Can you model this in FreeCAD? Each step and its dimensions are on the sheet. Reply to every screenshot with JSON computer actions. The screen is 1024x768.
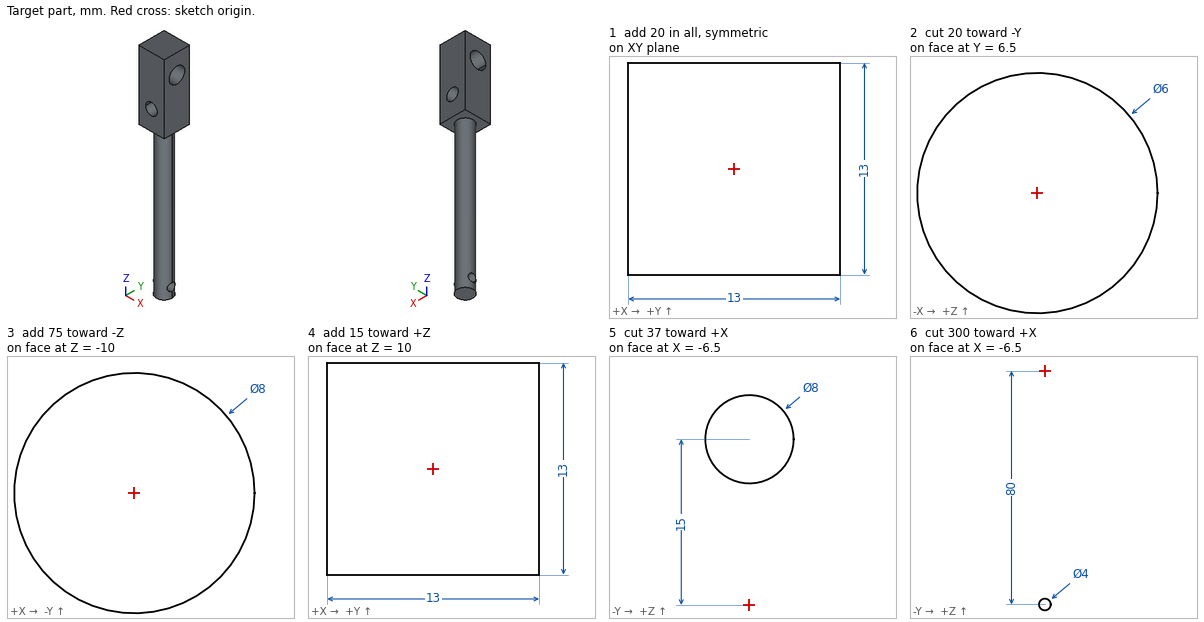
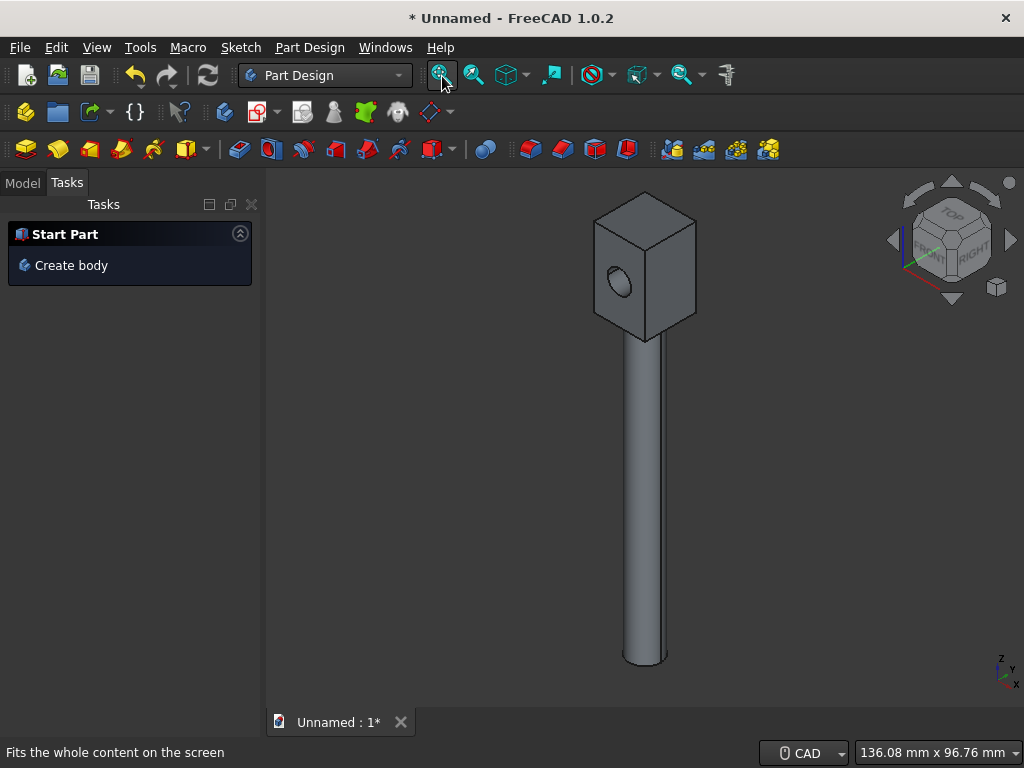
{"action": "left_click", "coordinate": [645, 220]}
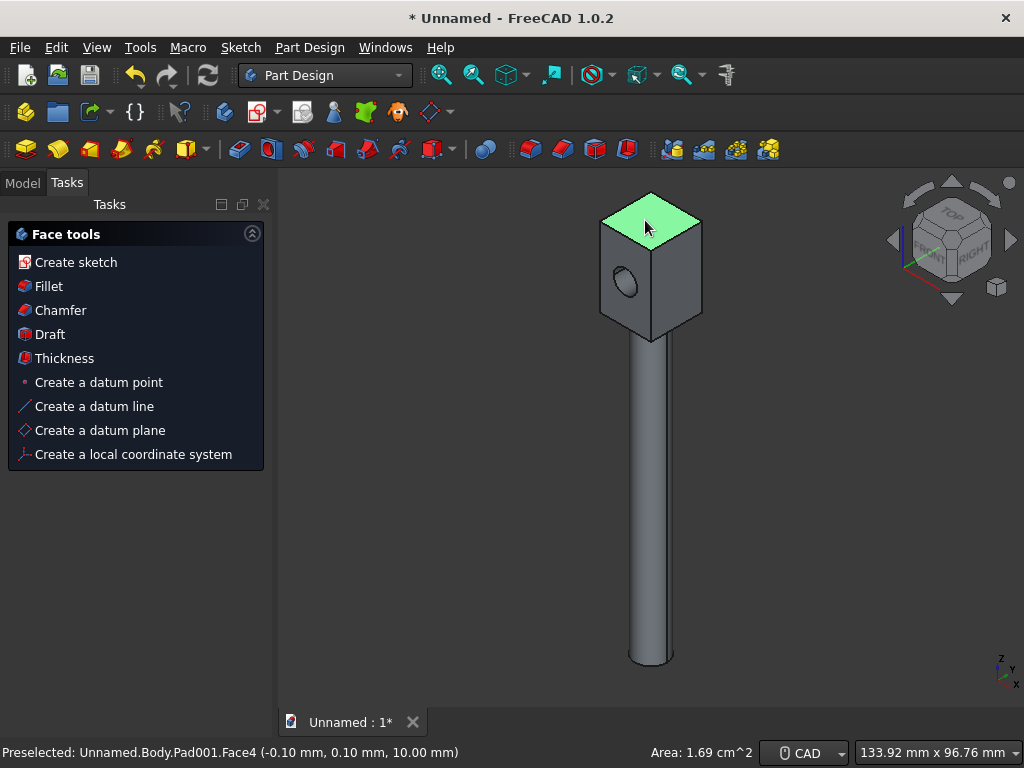
{"action": "left_click", "coordinate": [258, 112]}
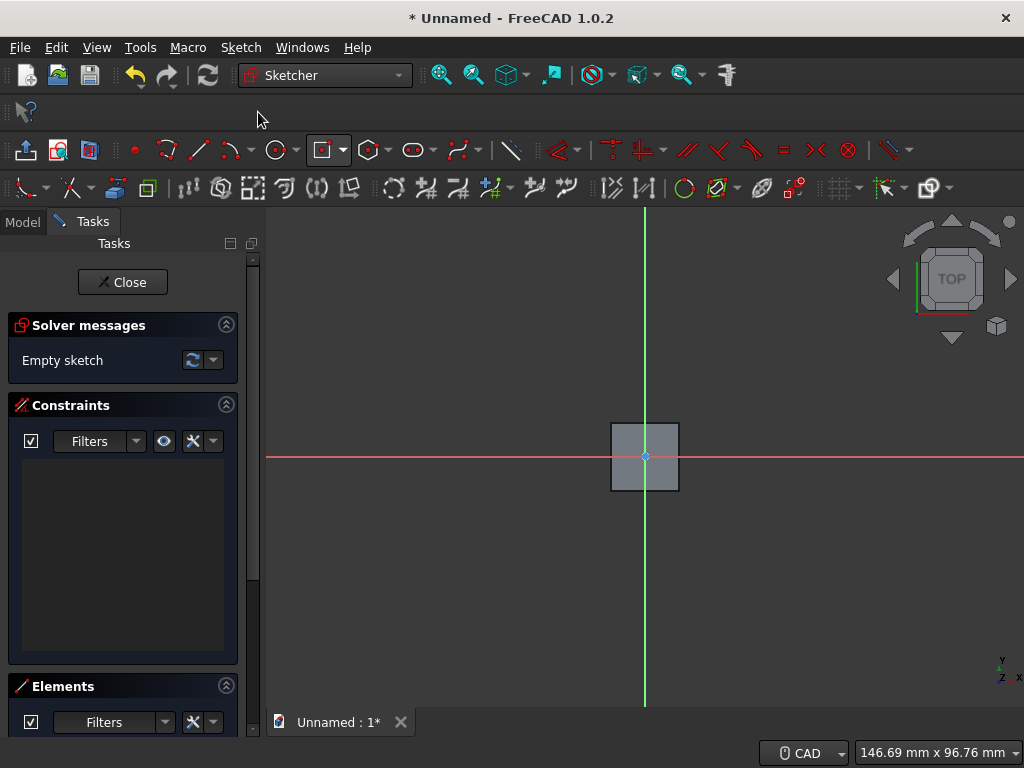
{"action": "scroll", "coordinate": [662, 457], "scroll_direction": "up", "scroll_amount": 8}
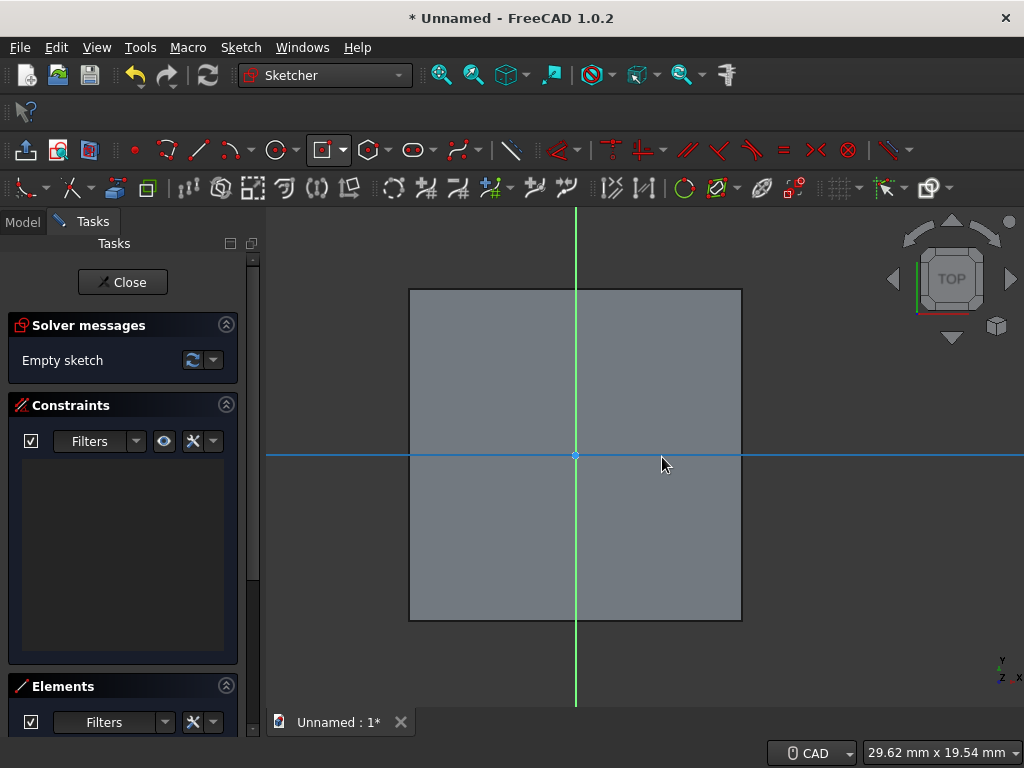
{"action": "left_click", "coordinate": [322, 150]}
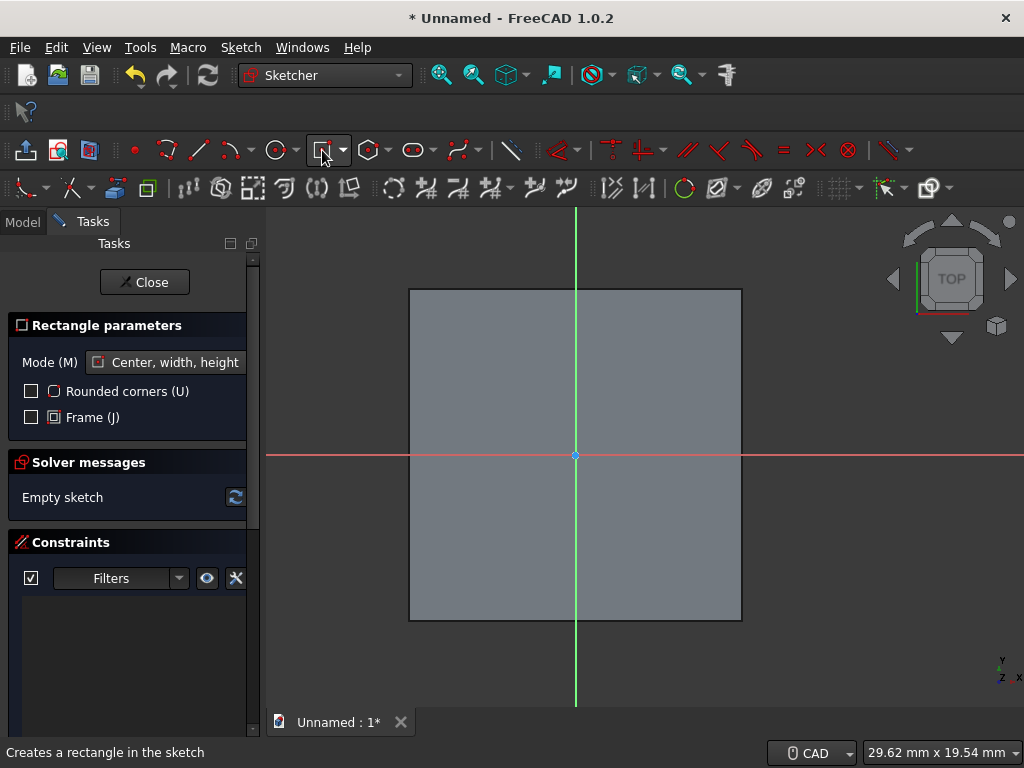
{"action": "left_click", "coordinate": [576, 455]}
{"action": "mouse_move", "coordinate": [742, 289]}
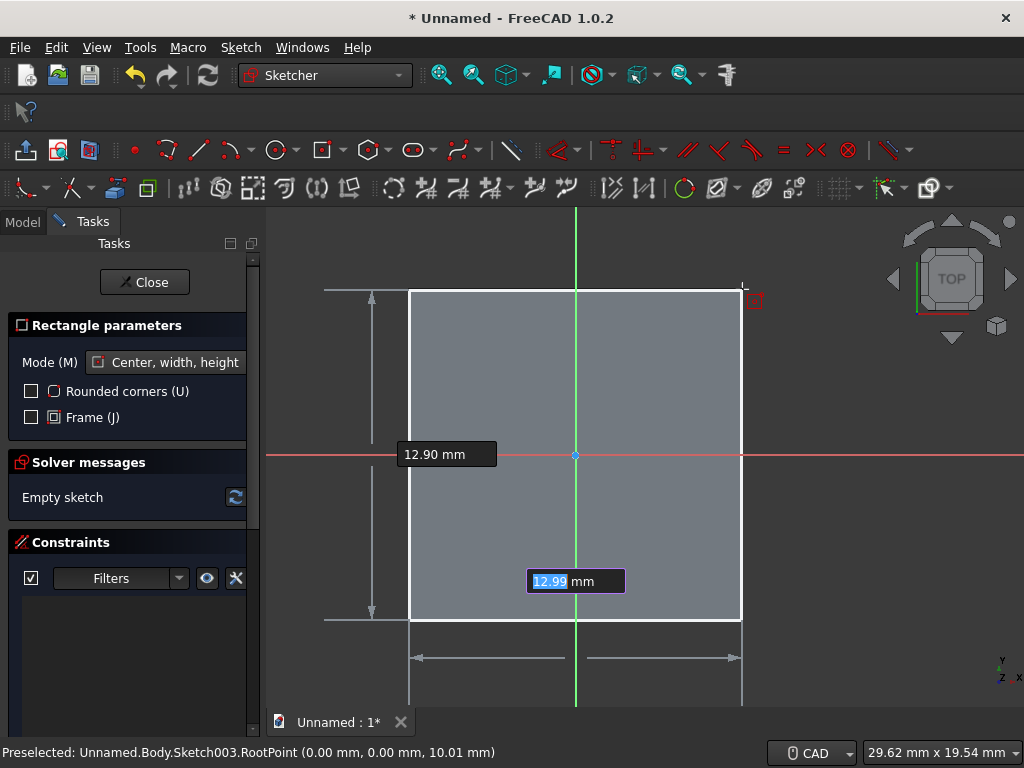
{"action": "type", "text": "13"}
{"action": "key", "text": "Tab"}
{"action": "type", "text": "13"}
{"action": "key", "text": "Return"}
{"action": "key", "text": "Escape"}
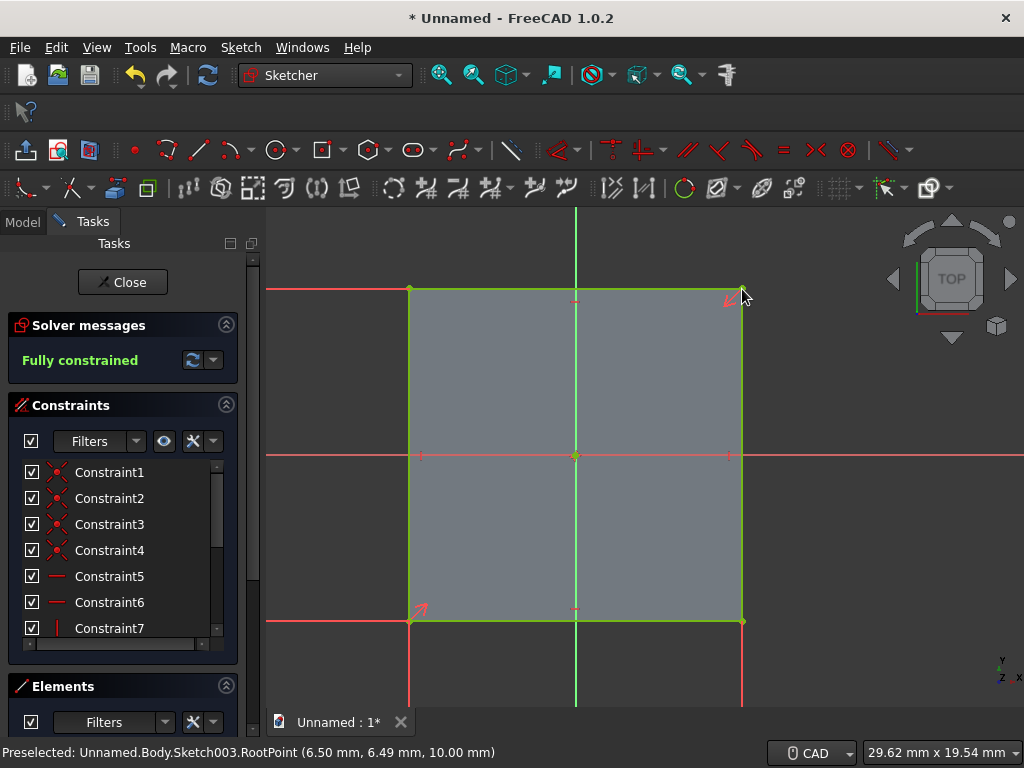
{"action": "left_click", "coordinate": [123, 282]}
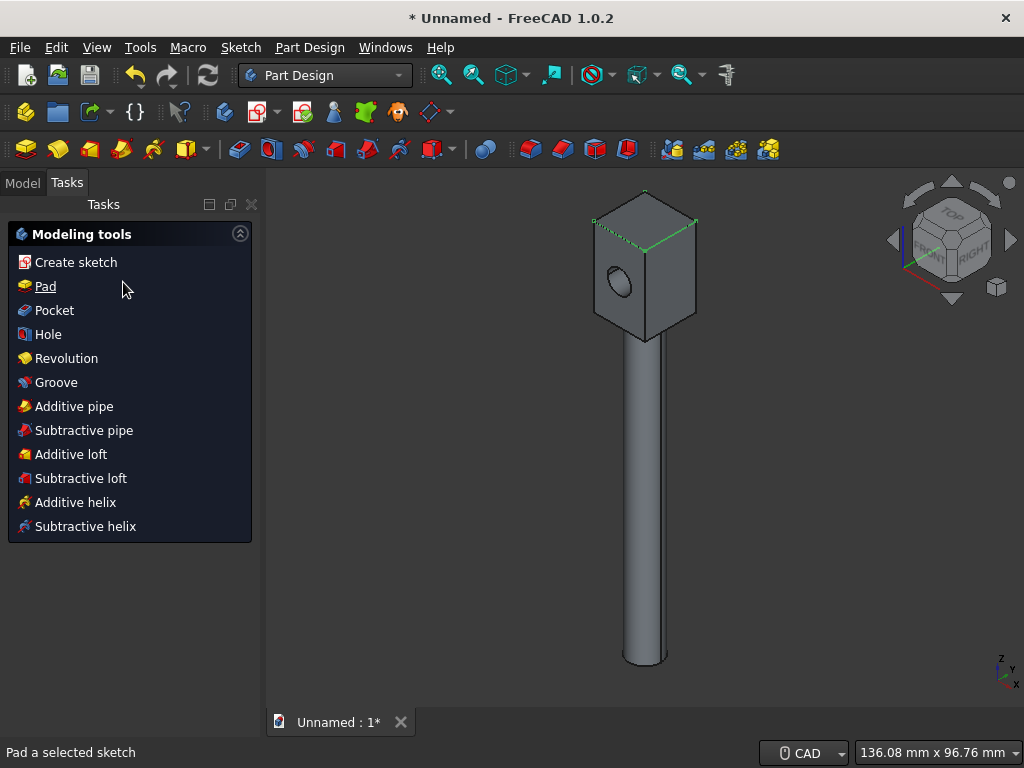
{"action": "left_click", "coordinate": [26, 150]}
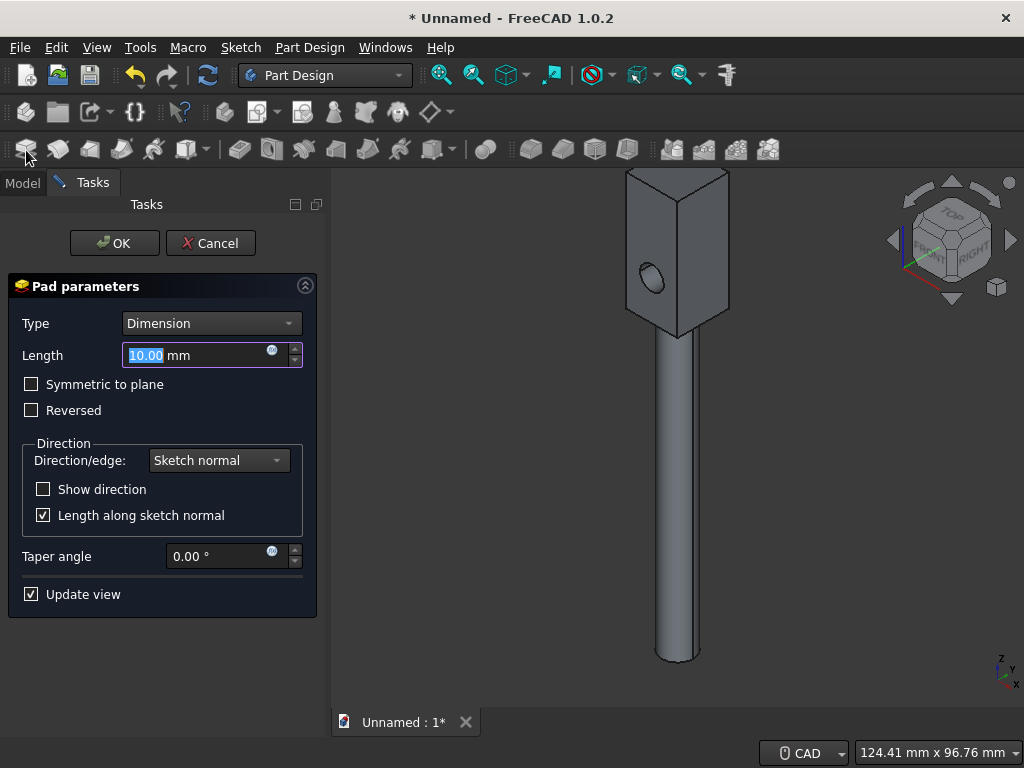
{"action": "type", "text": "15"}
{"action": "key", "text": "Tab"}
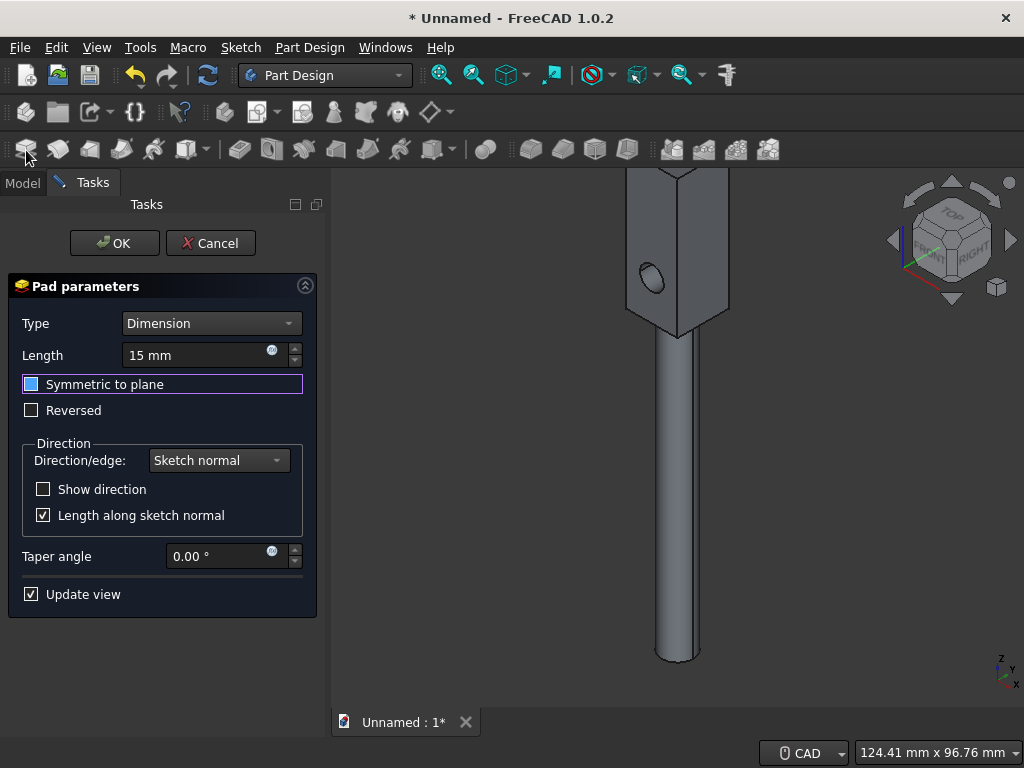
{"action": "left_click", "coordinate": [115, 243]}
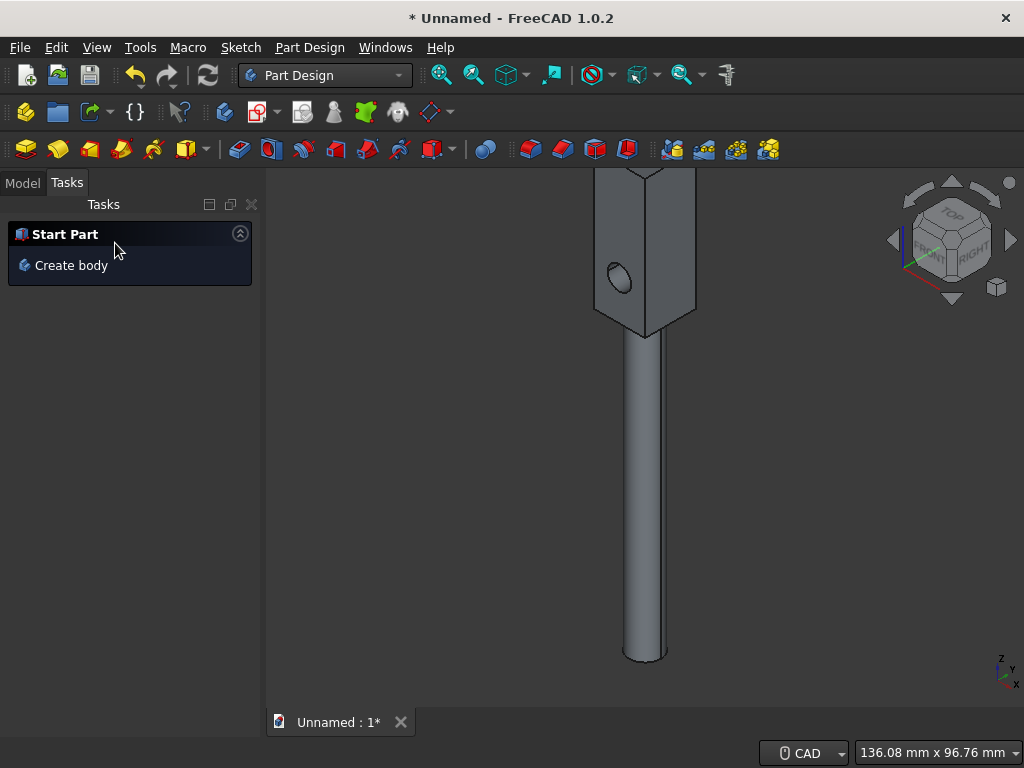
{"action": "left_click", "coordinate": [442, 76]}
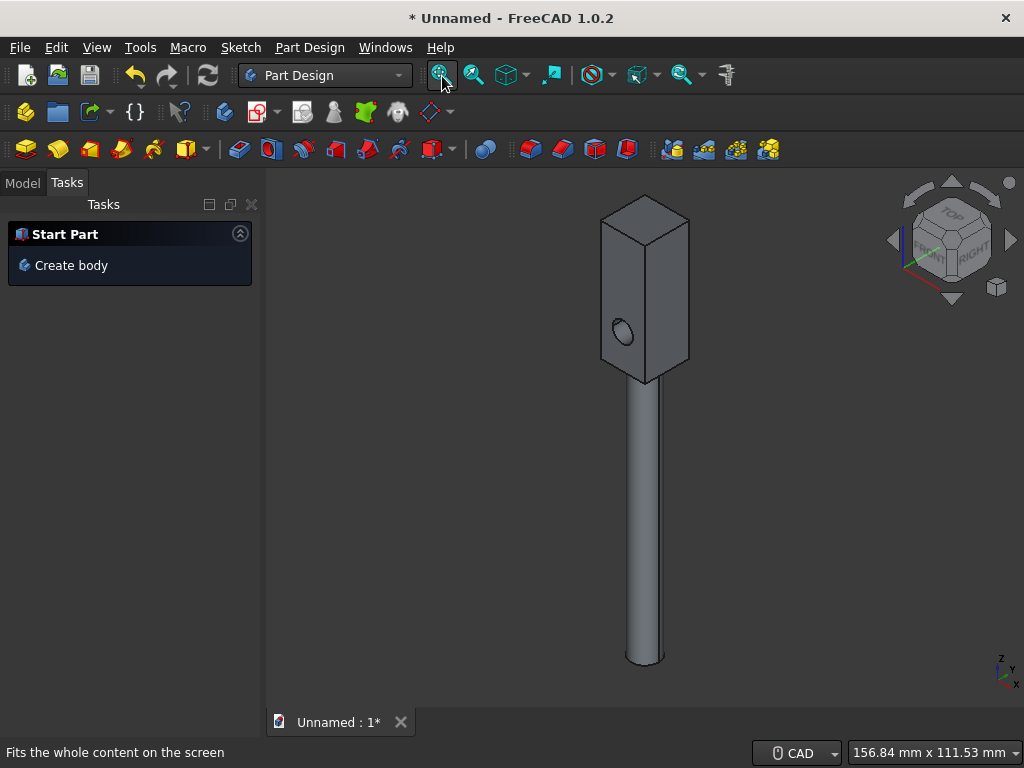
{"action": "key", "text": "6"}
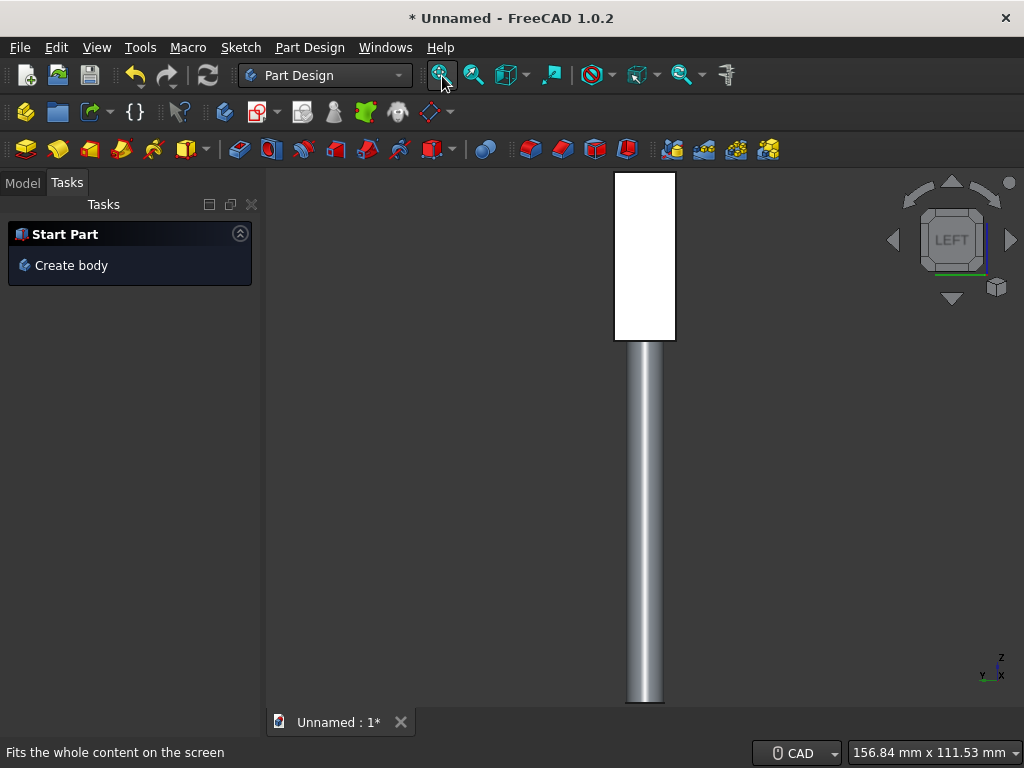
{"action": "left_click", "coordinate": [645, 207]}